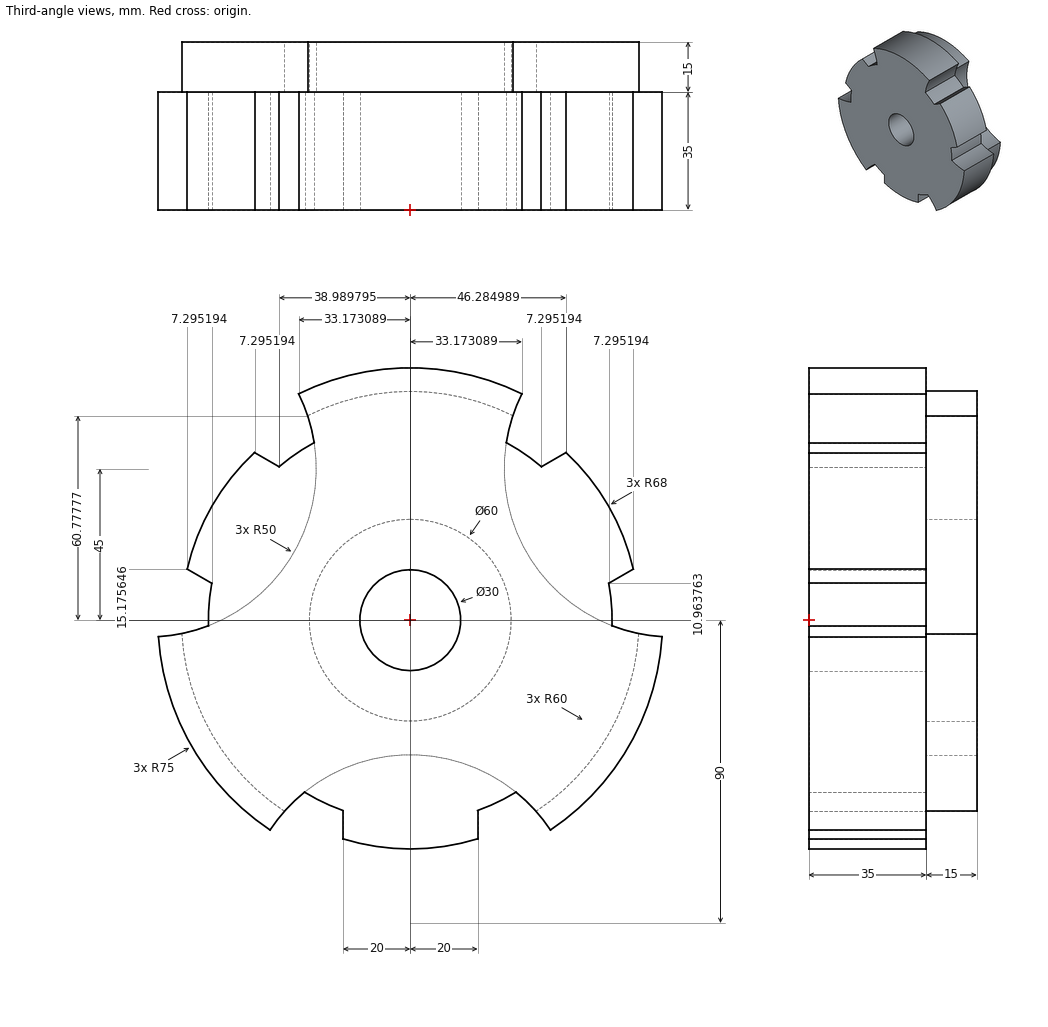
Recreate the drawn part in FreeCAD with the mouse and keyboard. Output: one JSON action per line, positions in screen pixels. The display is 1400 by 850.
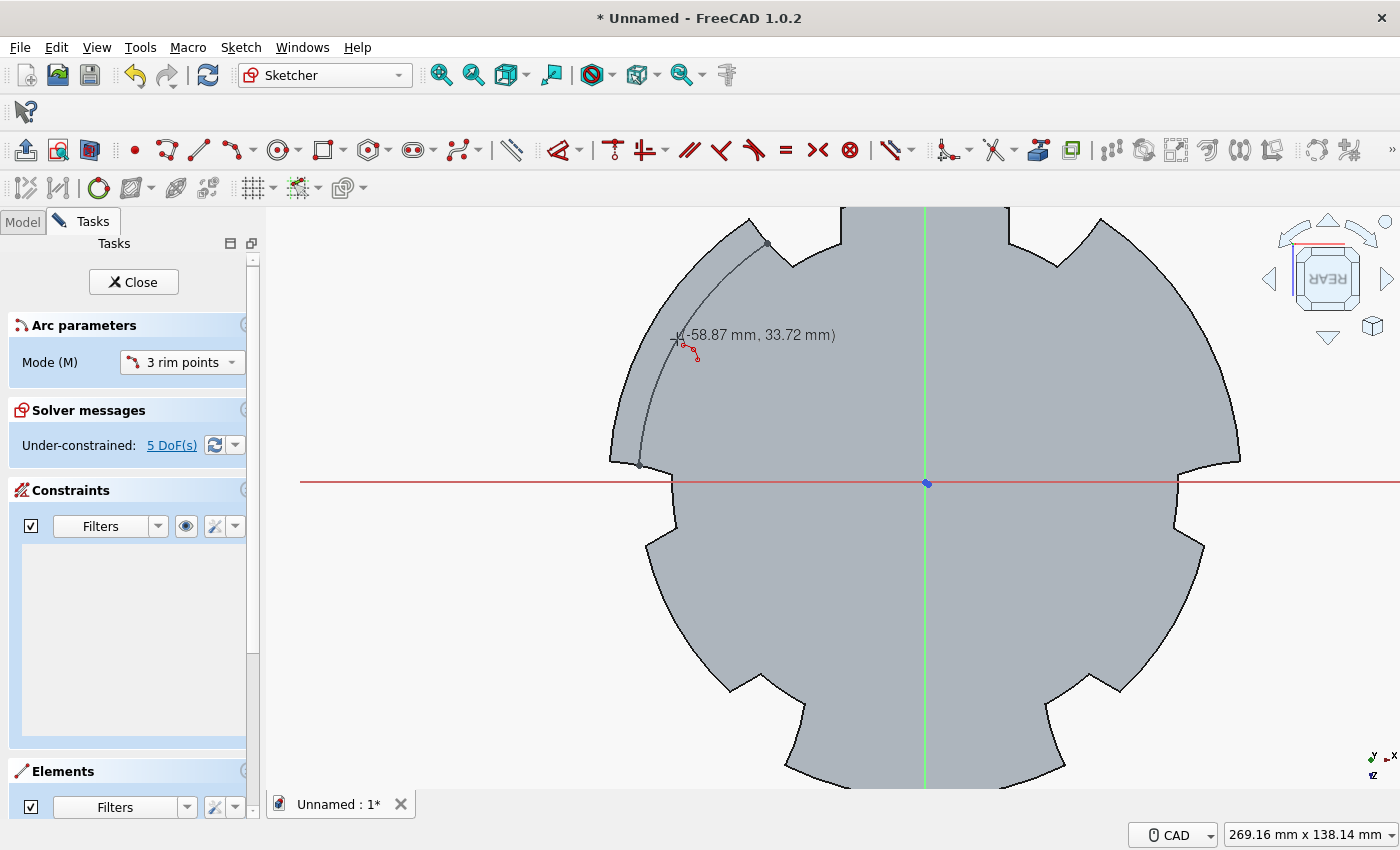
{"action": "left_click", "coordinate": [639, 466]}
{"action": "left_click", "coordinate": [797, 738]}
{"action": "left_click", "coordinate": [779, 566]}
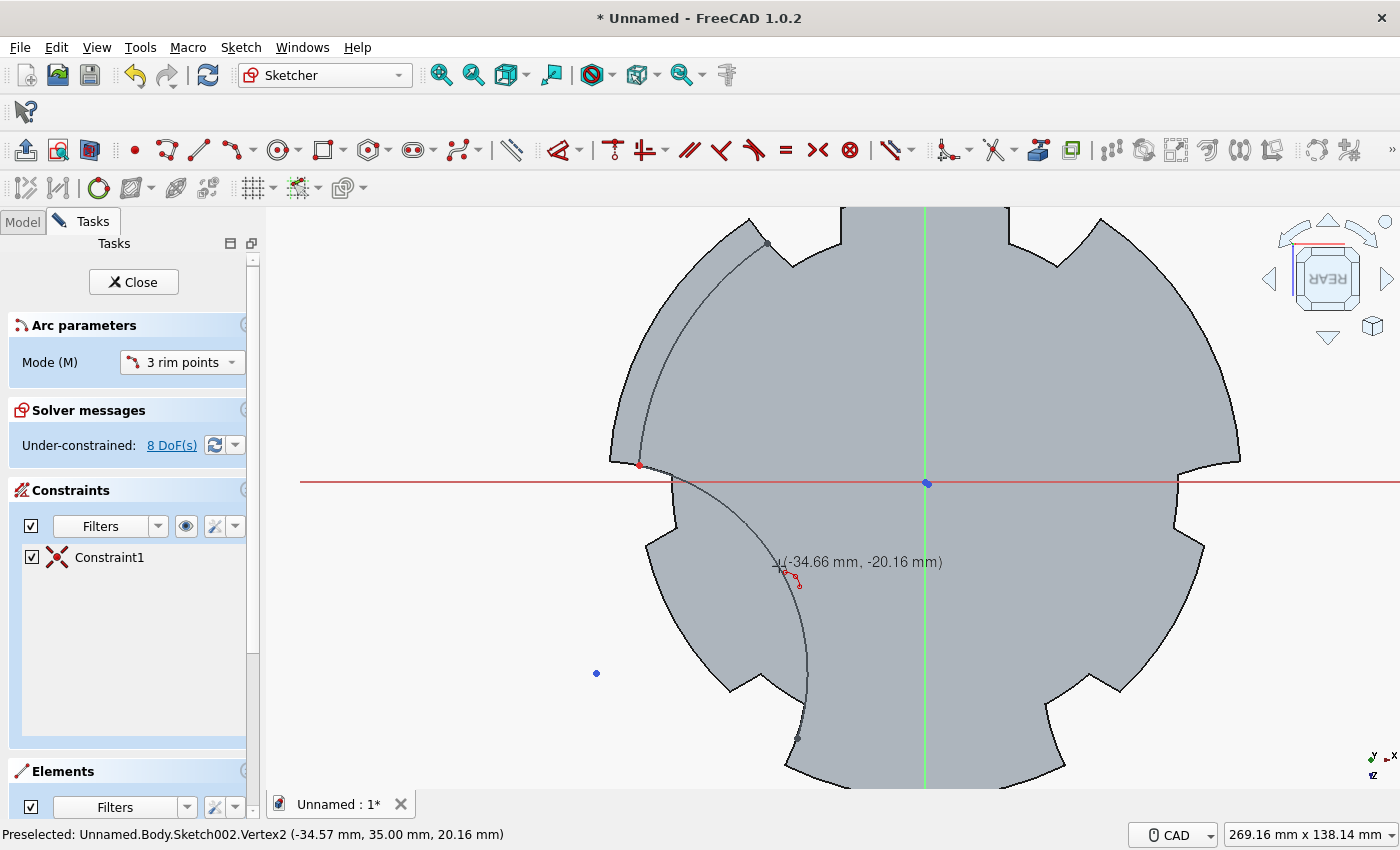
{"action": "left_click", "coordinate": [797, 739]}
{"action": "left_click", "coordinate": [1054, 738]}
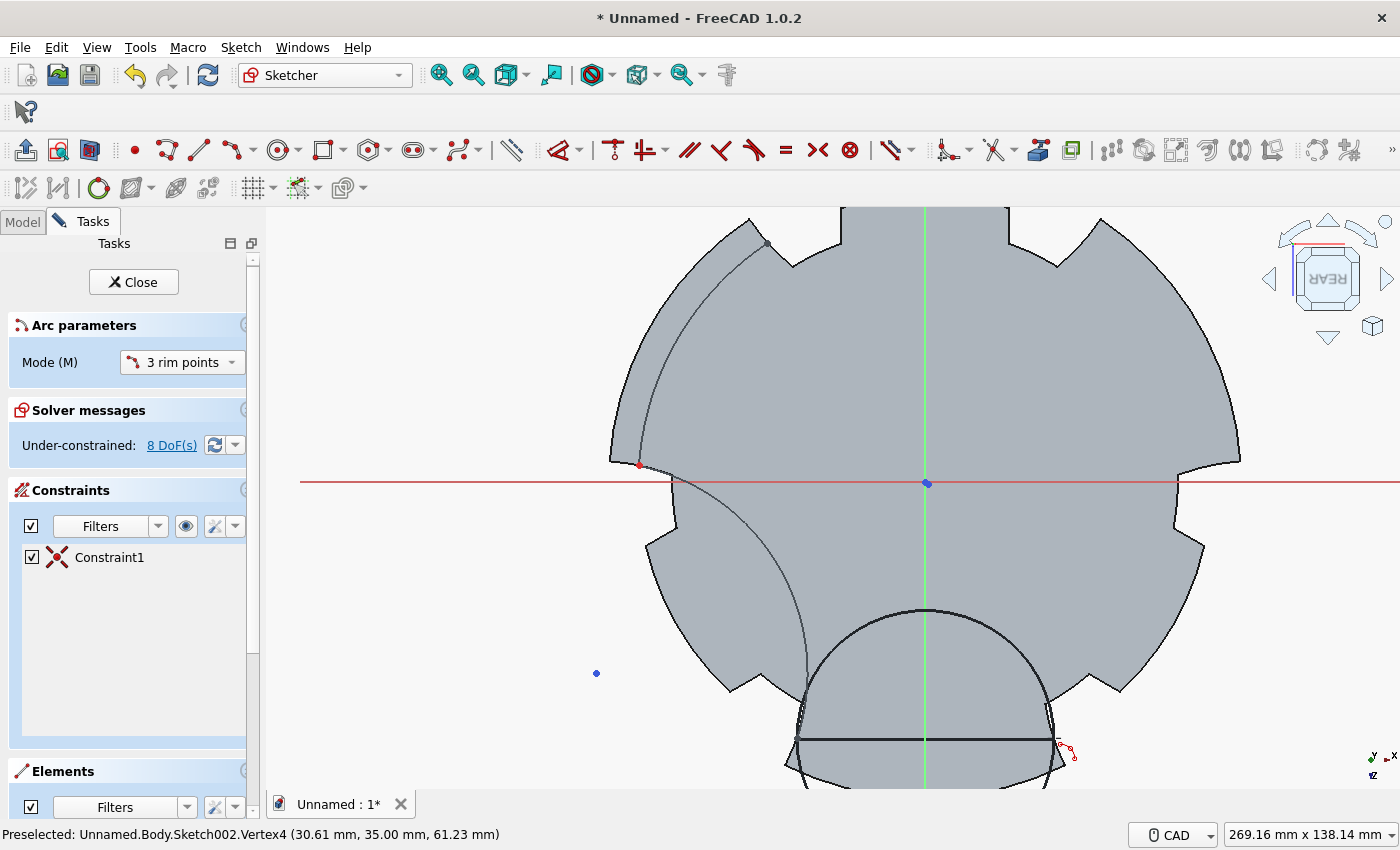
{"action": "scroll", "coordinate": [438, 482], "scroll_direction": "down", "scroll_amount": 2}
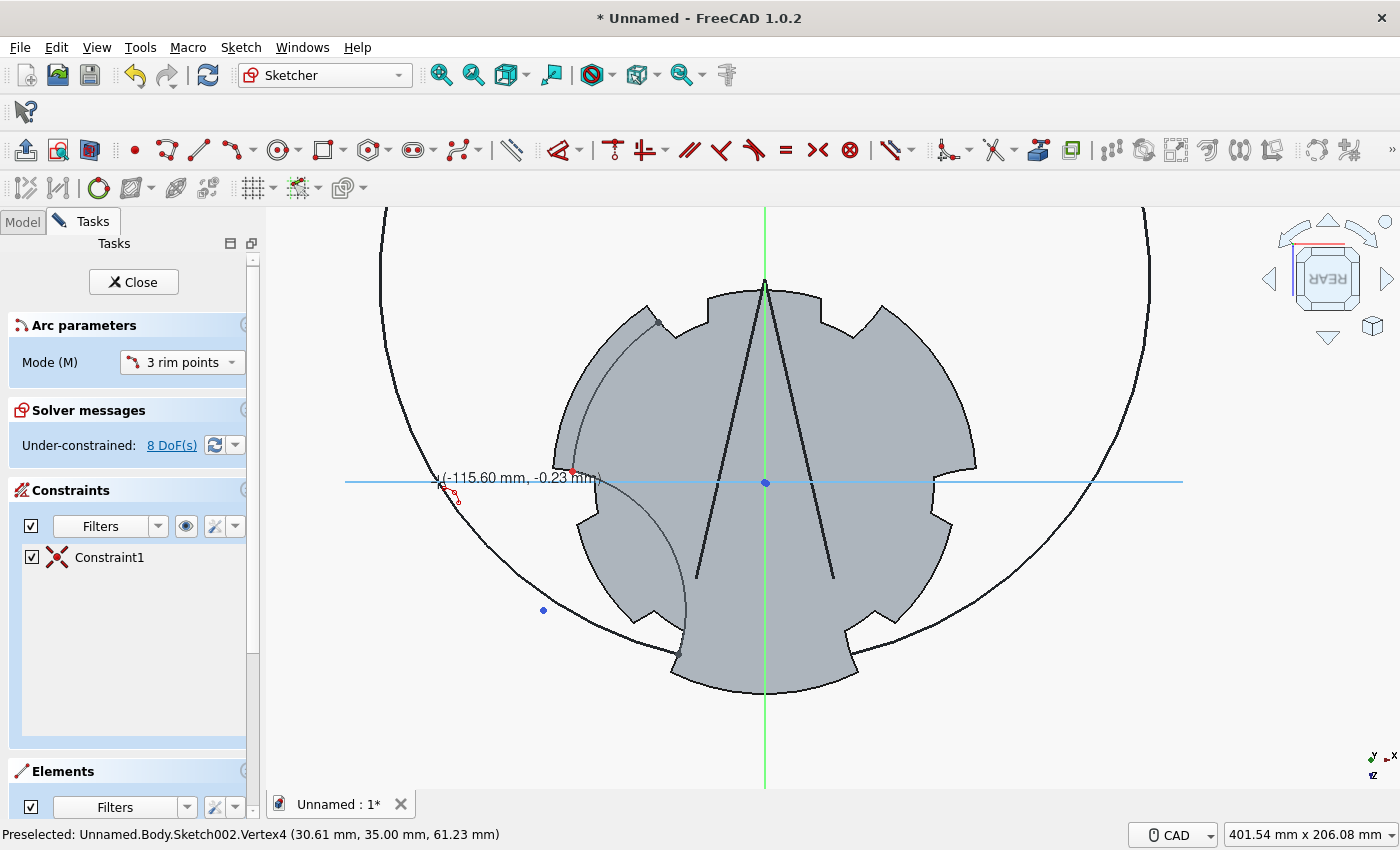
{"action": "left_click", "coordinate": [747, 673]}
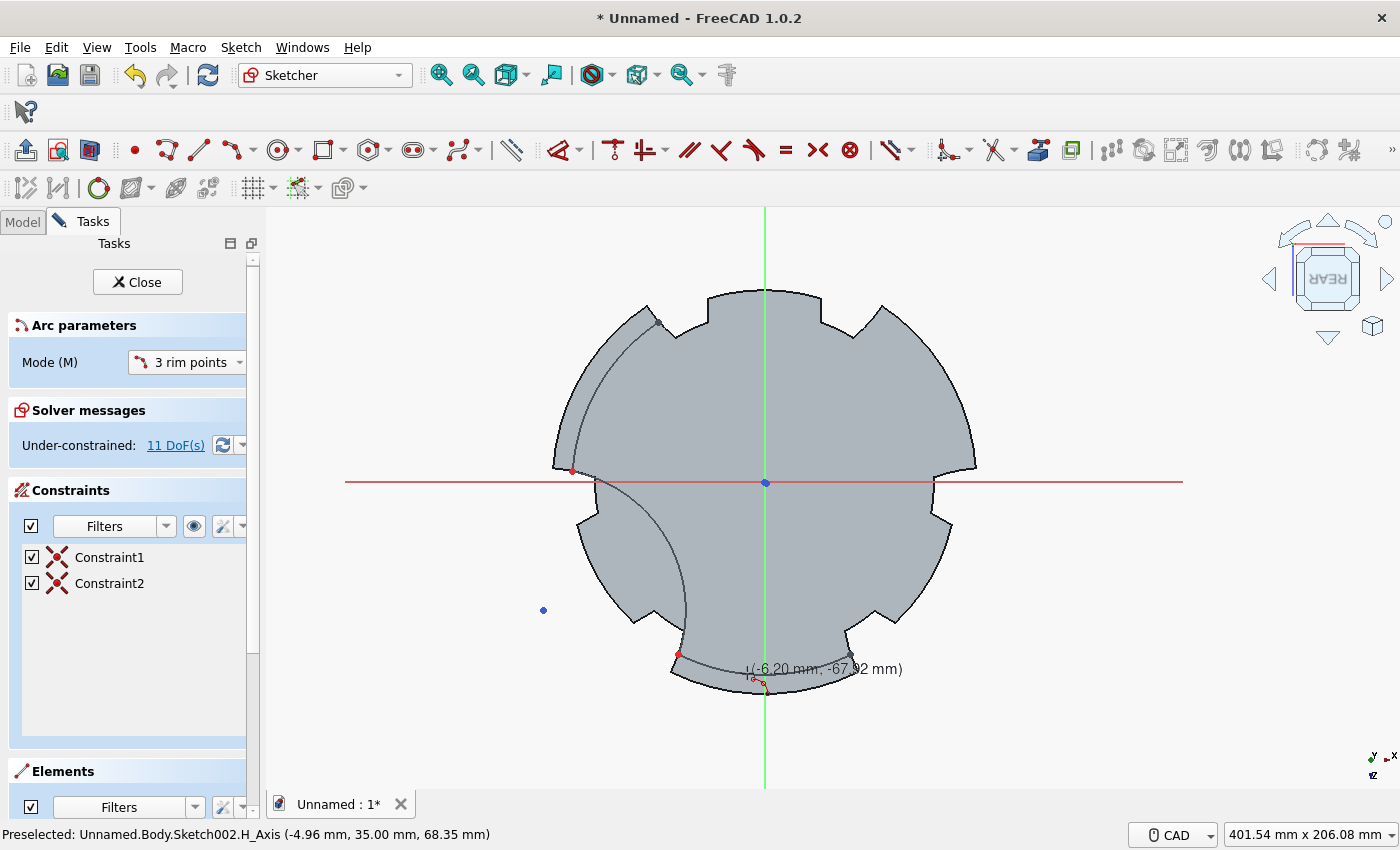
{"action": "left_click", "coordinate": [851, 654]}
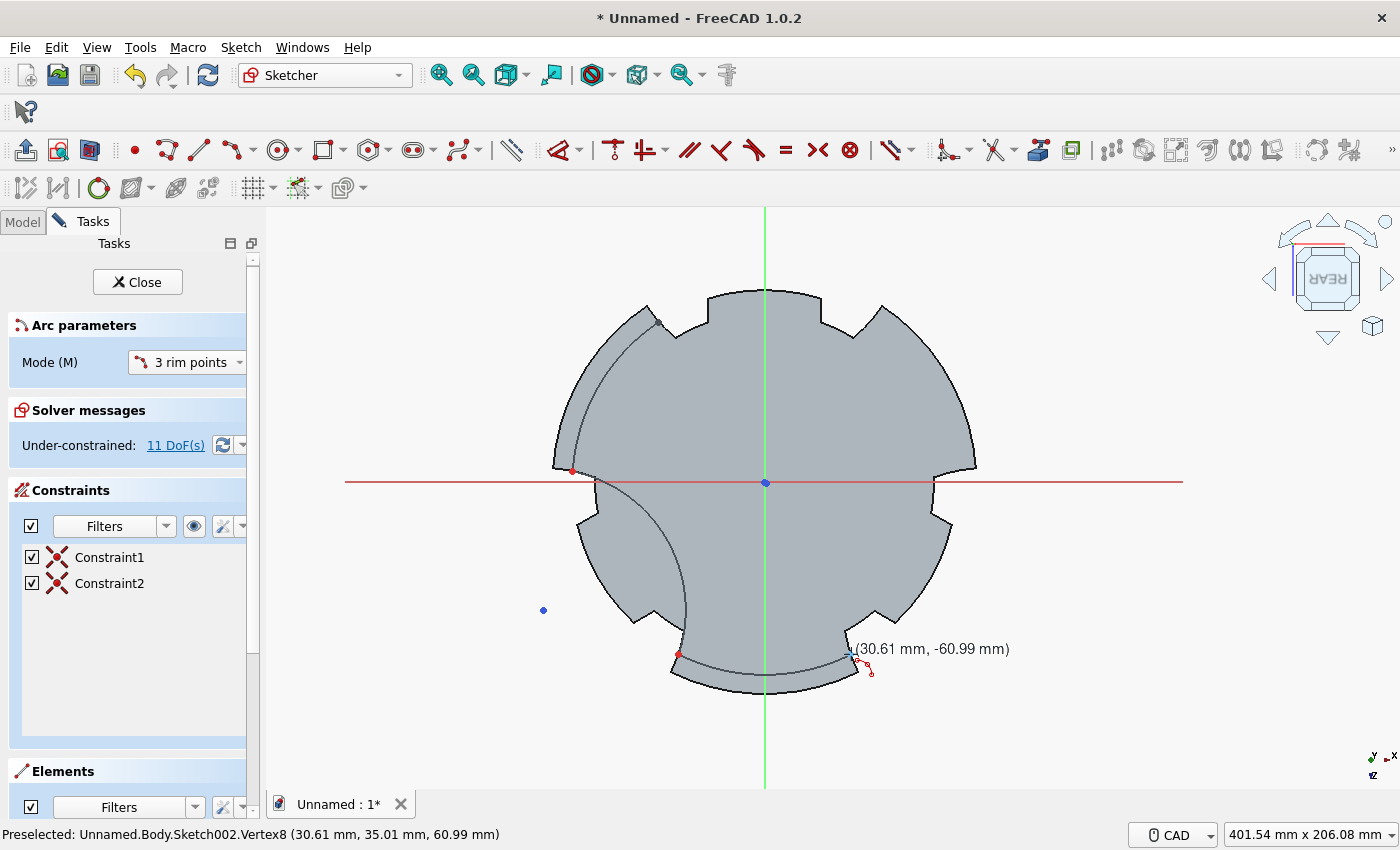
{"action": "scroll", "coordinate": [956, 471], "scroll_direction": "up", "scroll_amount": 2}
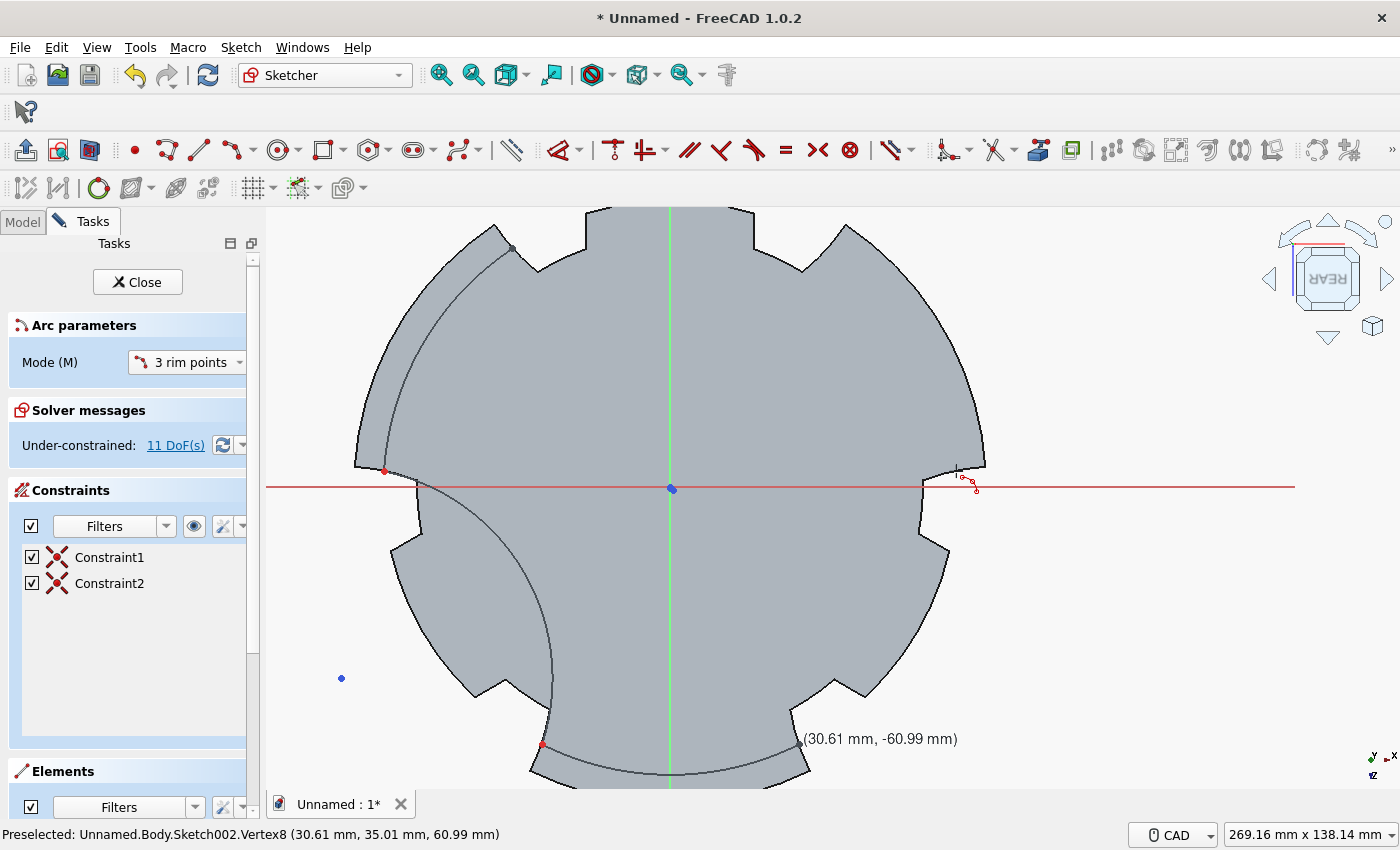
{"action": "left_click", "coordinate": [956, 471]}
{"action": "left_click", "coordinate": [816, 572]}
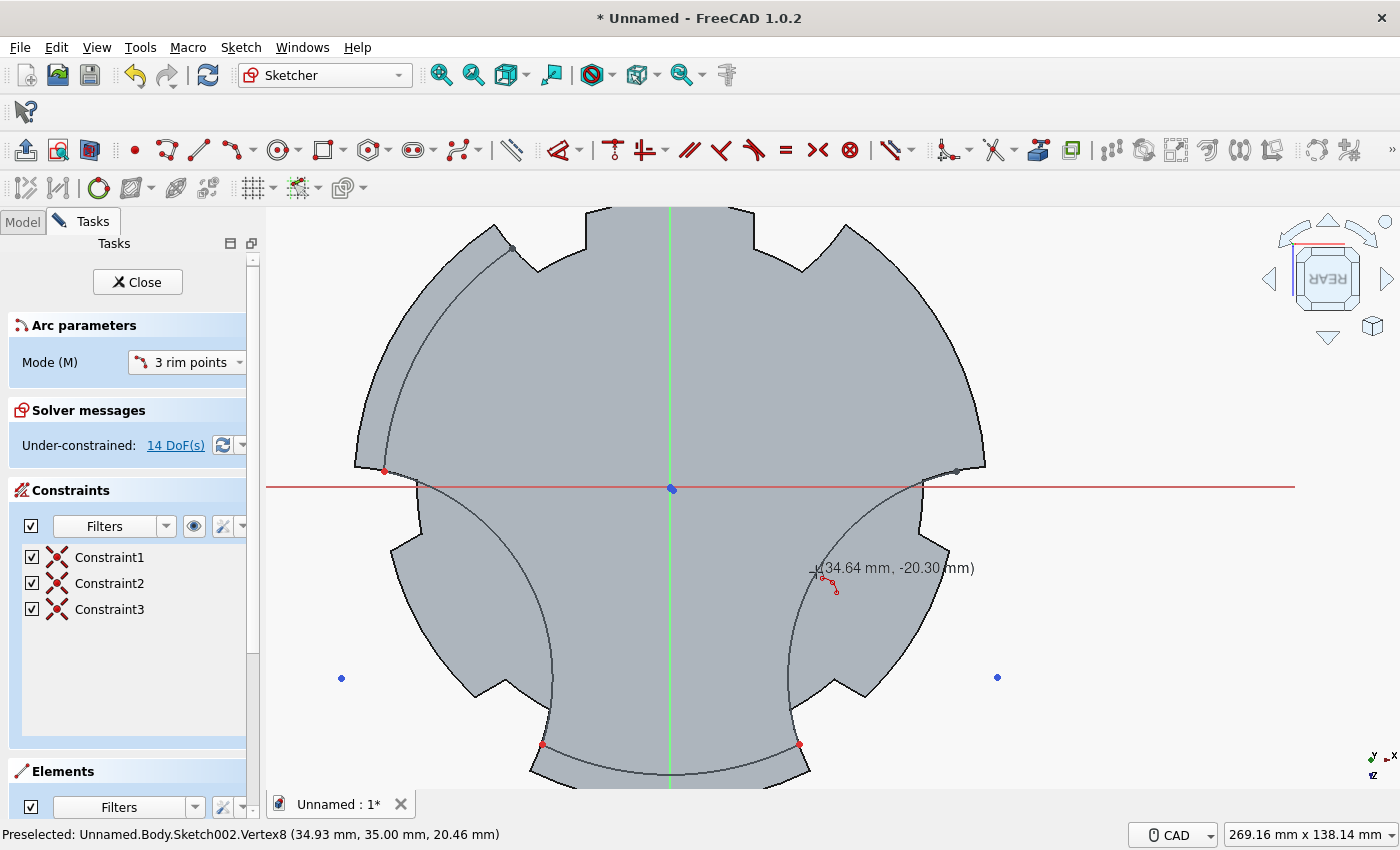
{"action": "left_click", "coordinate": [956, 472]}
{"action": "left_click", "coordinate": [828, 248]}
{"action": "left_click", "coordinate": [918, 344]}